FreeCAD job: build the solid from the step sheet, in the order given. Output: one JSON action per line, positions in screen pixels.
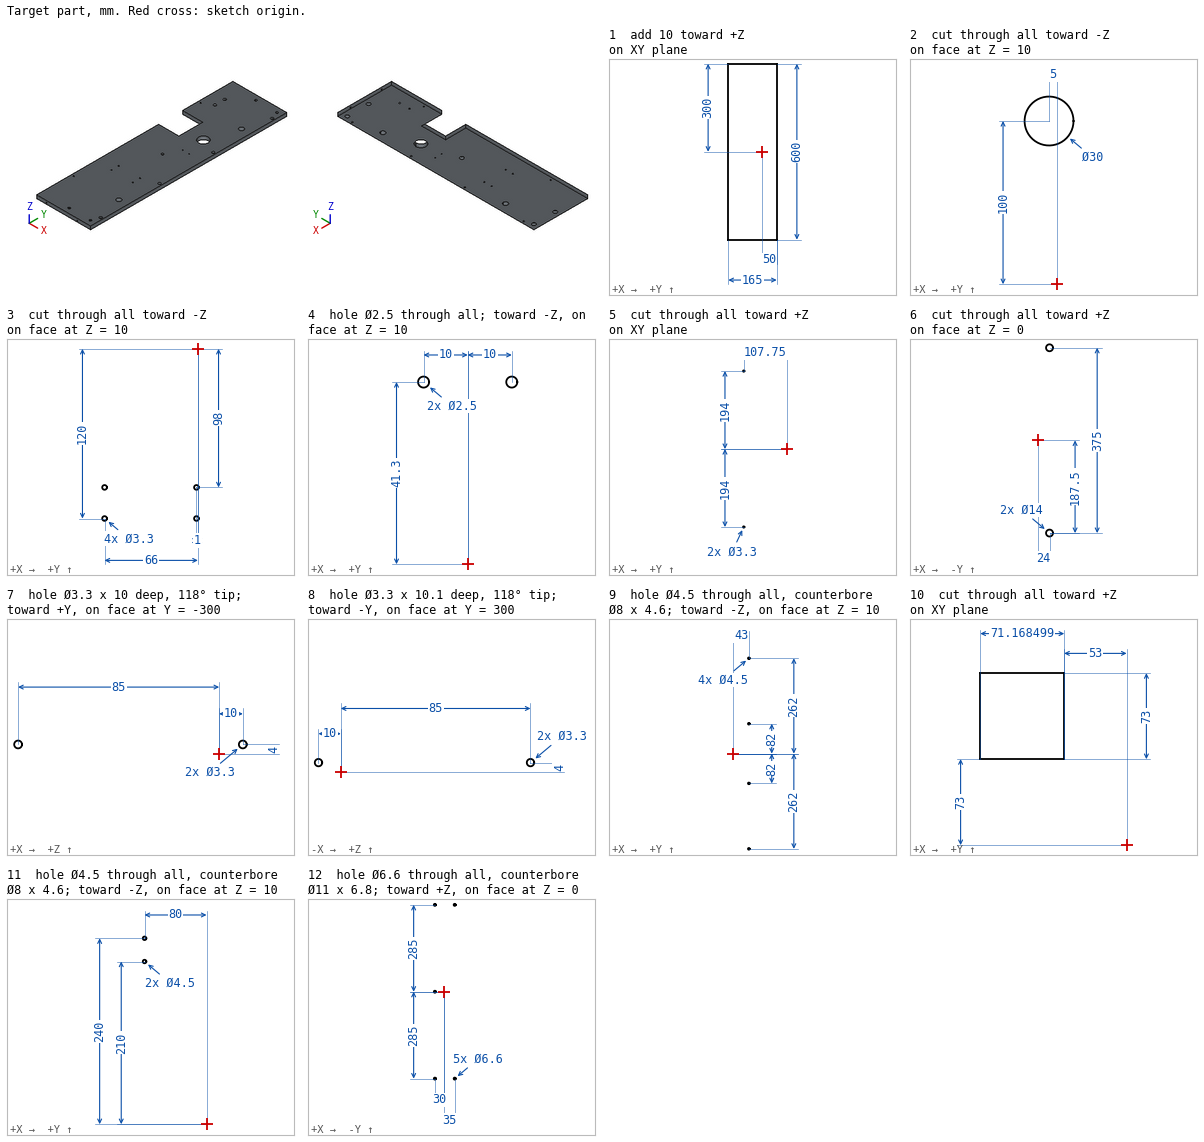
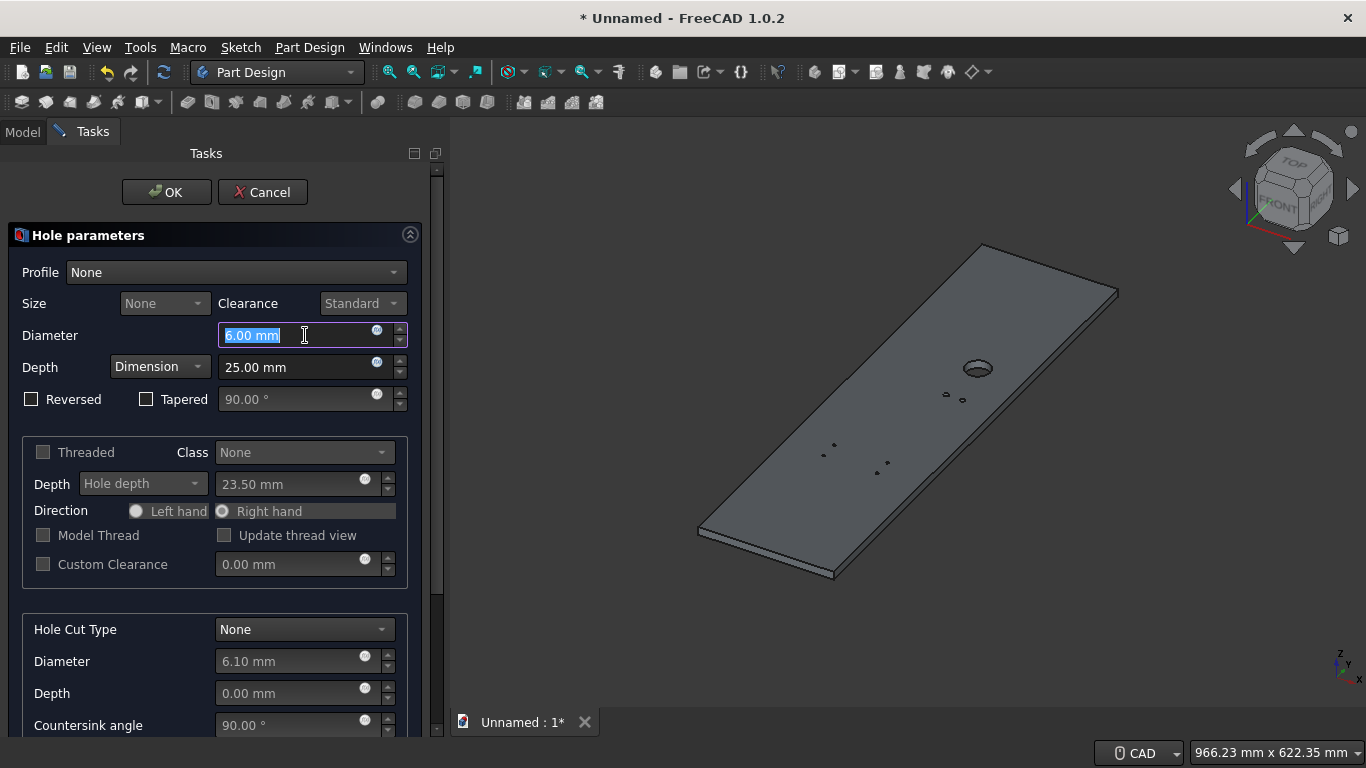
{"action": "type", "text": "2.5"}
{"action": "key", "text": "Tab"}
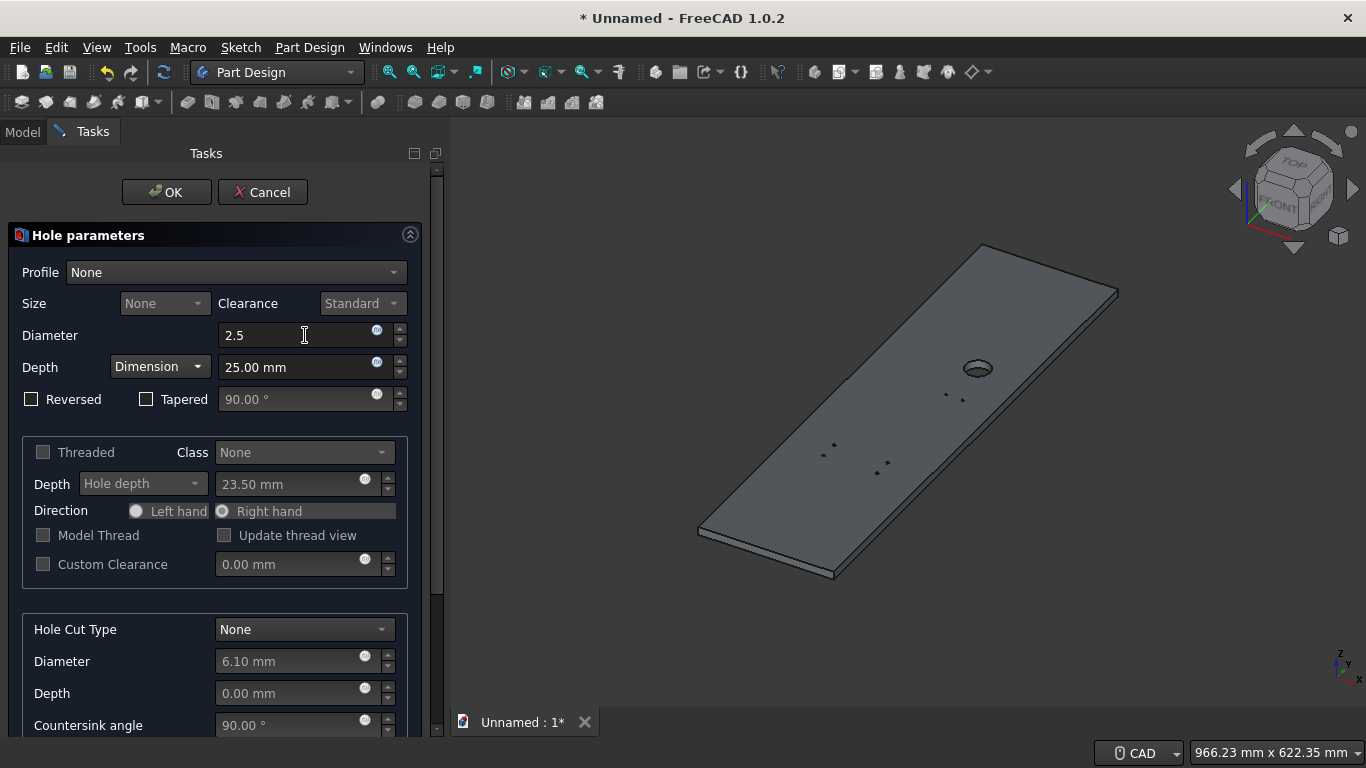
{"action": "left_click", "coordinate": [161, 366]}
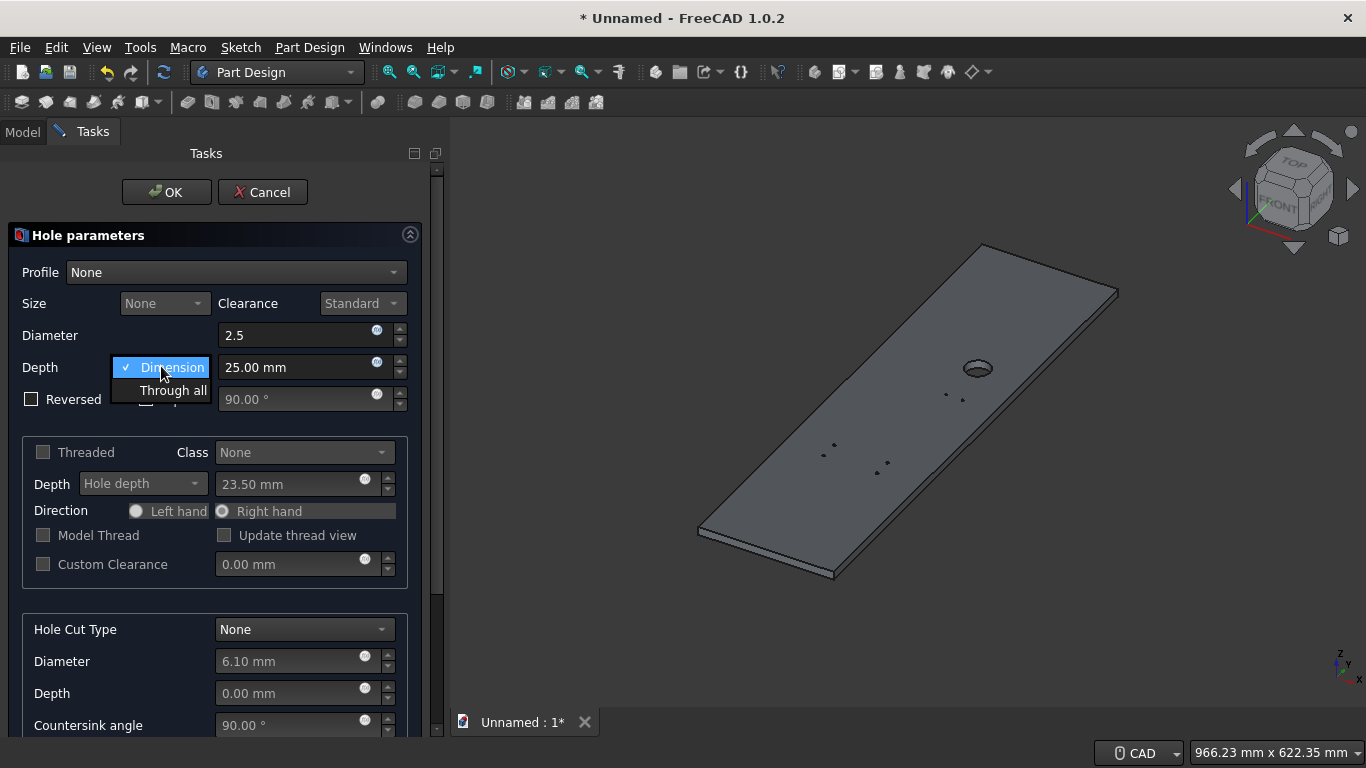
{"action": "left_click", "coordinate": [160, 390]}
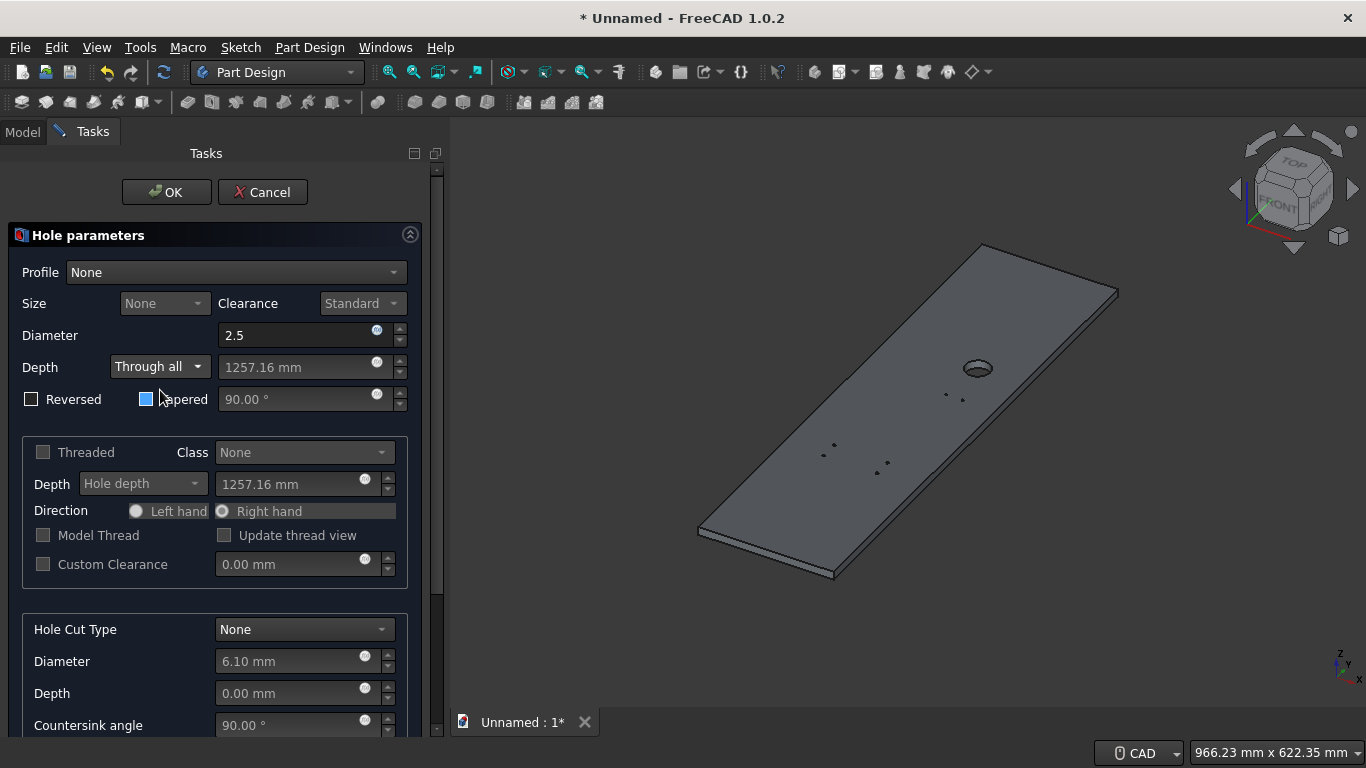
{"action": "left_click", "coordinate": [167, 192]}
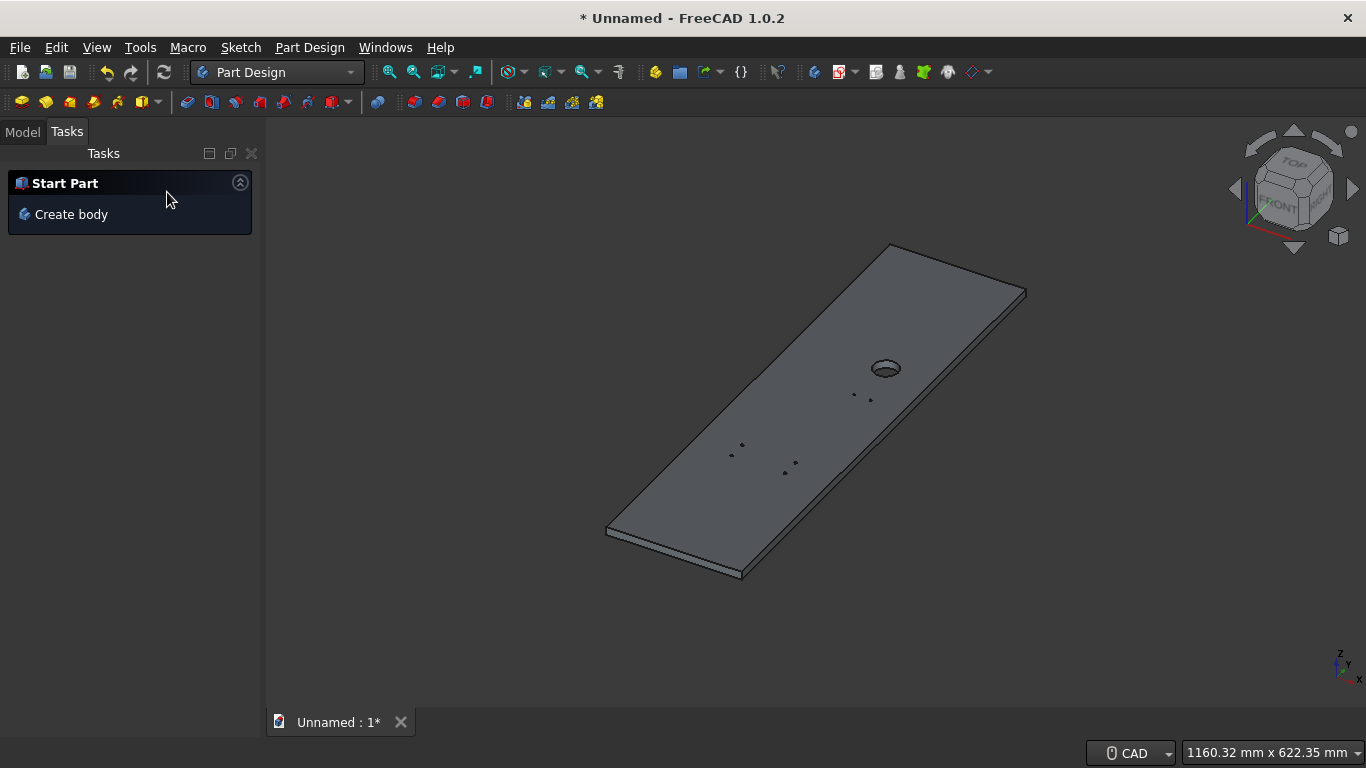
{"action": "left_click", "coordinate": [840, 72]}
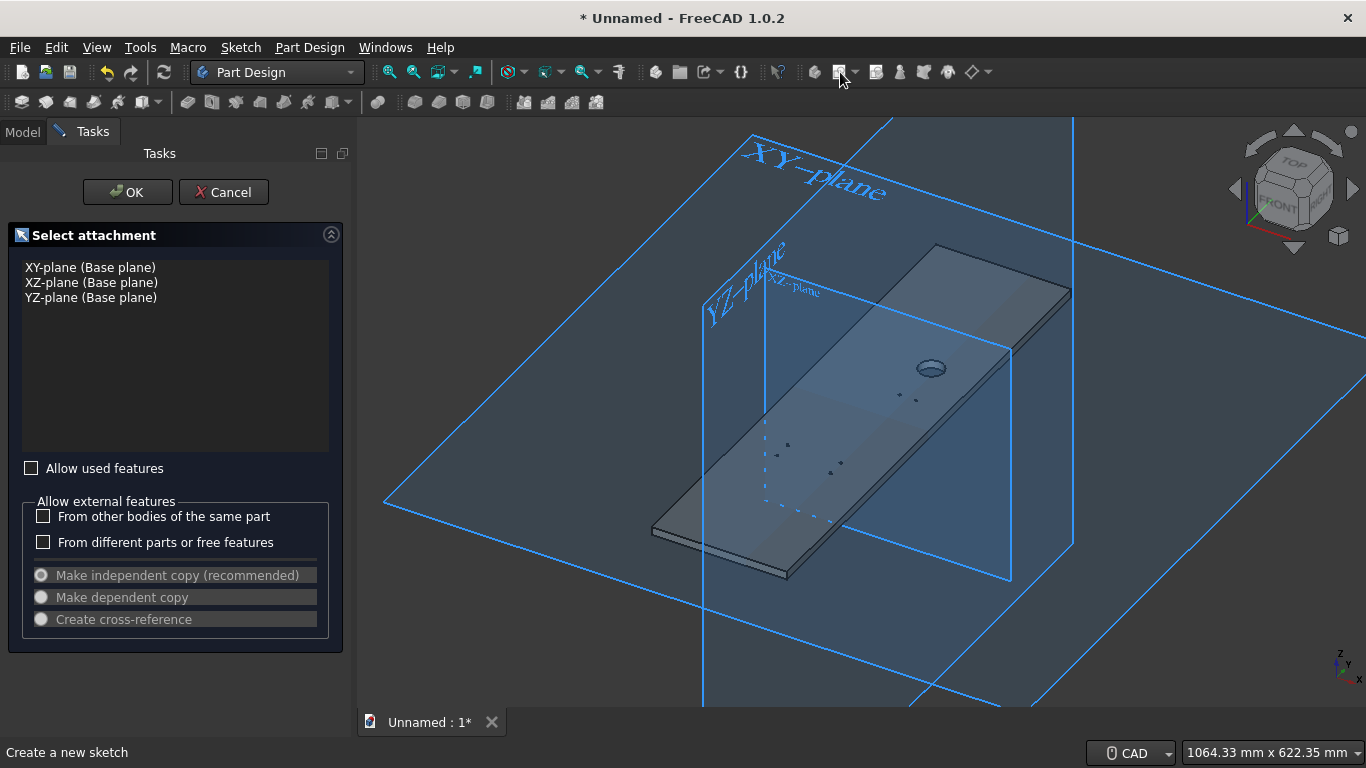
{"action": "left_click", "coordinate": [82, 268]}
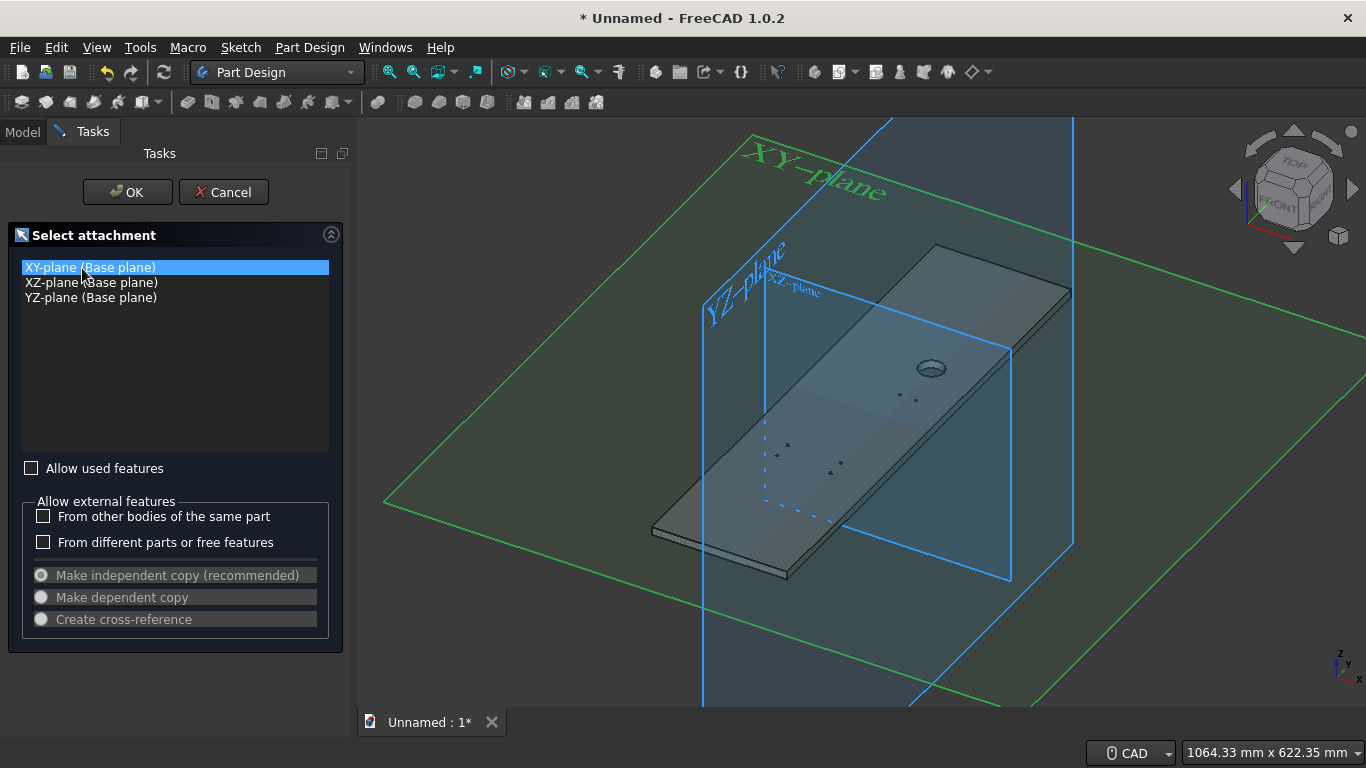
{"action": "left_click", "coordinate": [128, 192]}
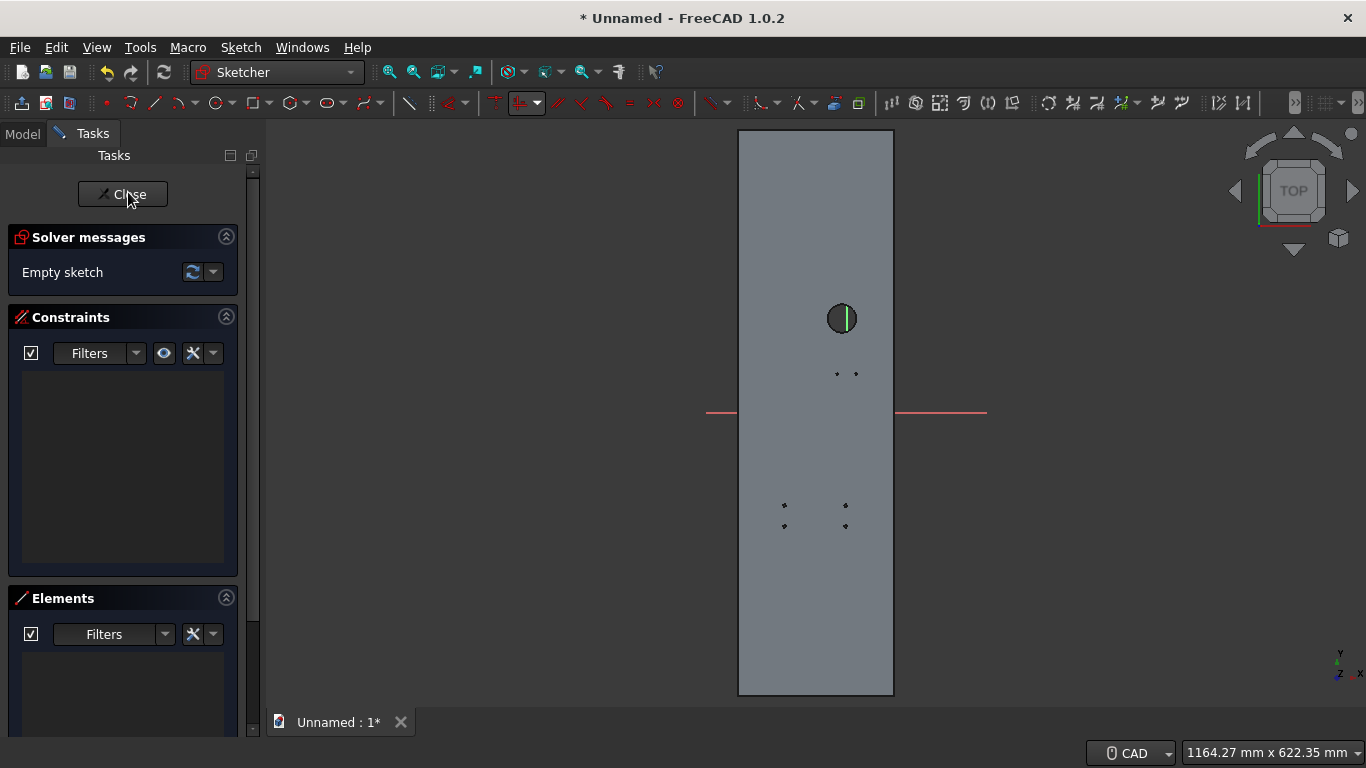
{"action": "left_click", "coordinate": [70, 104]}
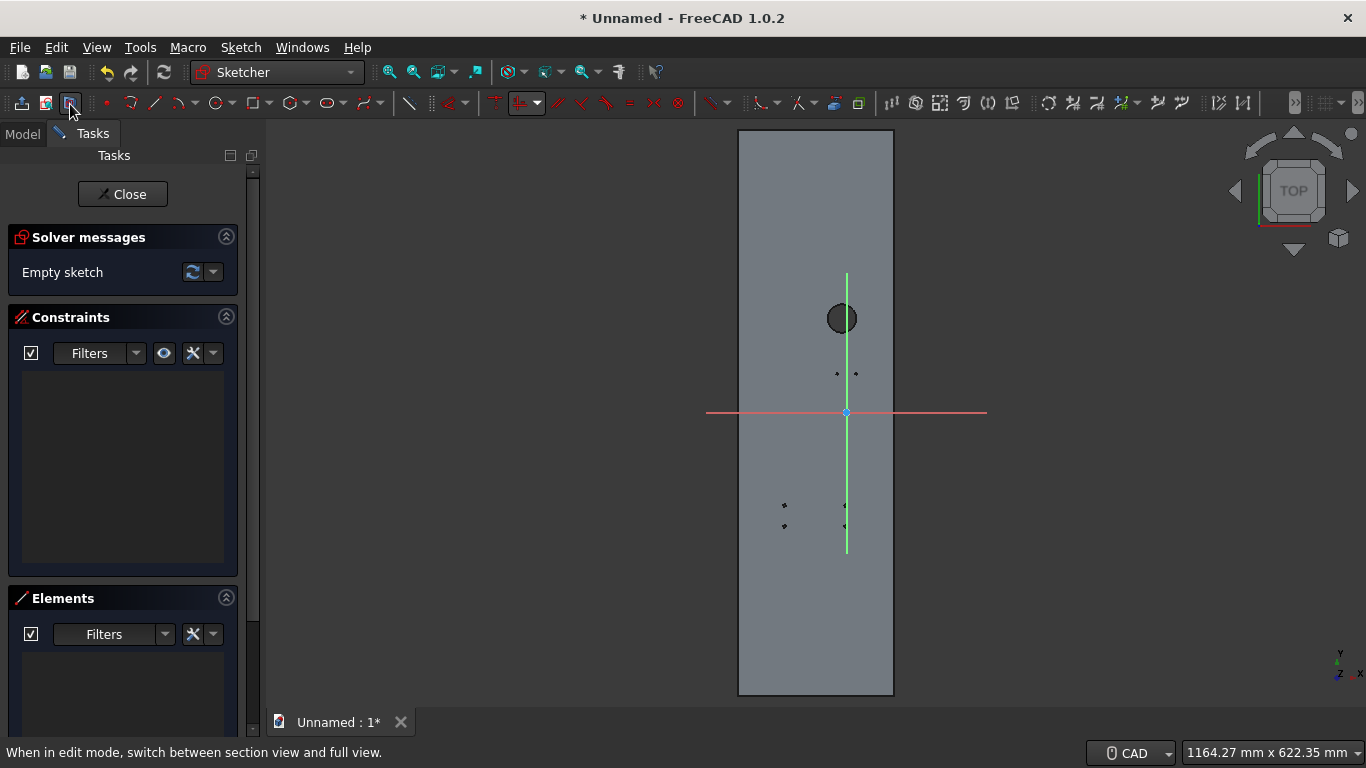
{"action": "left_click", "coordinate": [216, 104]}